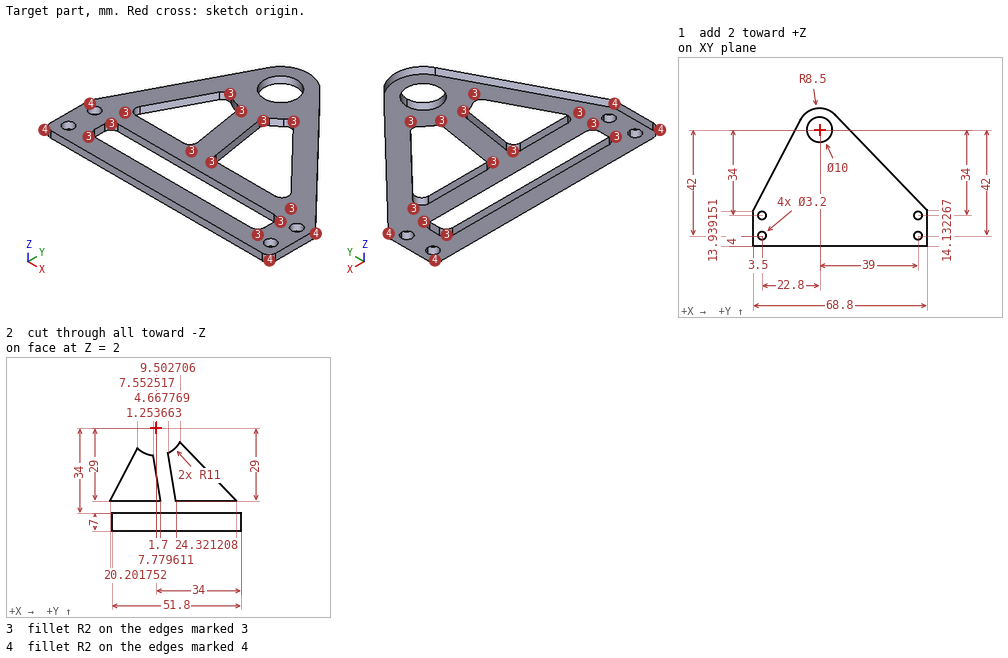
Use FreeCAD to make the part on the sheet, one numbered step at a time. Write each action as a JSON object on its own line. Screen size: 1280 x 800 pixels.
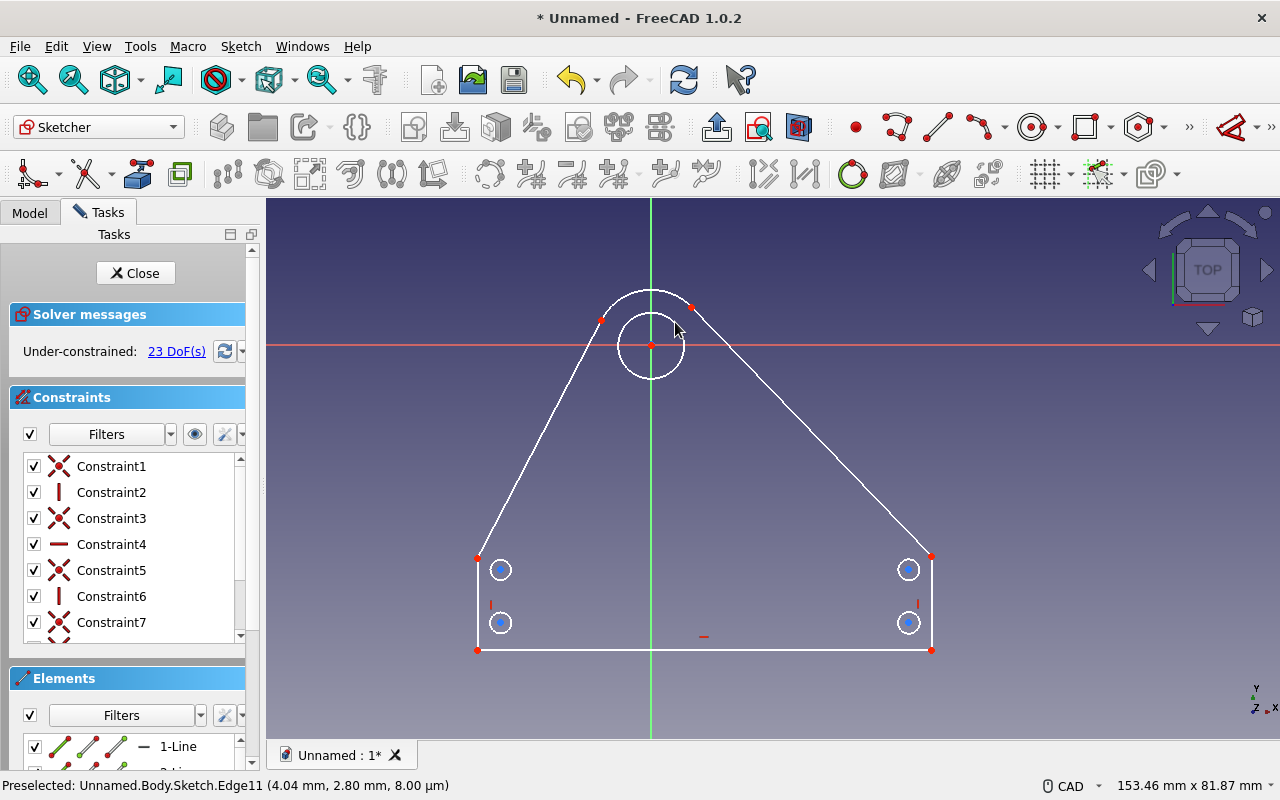
{"action": "left_click", "coordinate": [564, 392]}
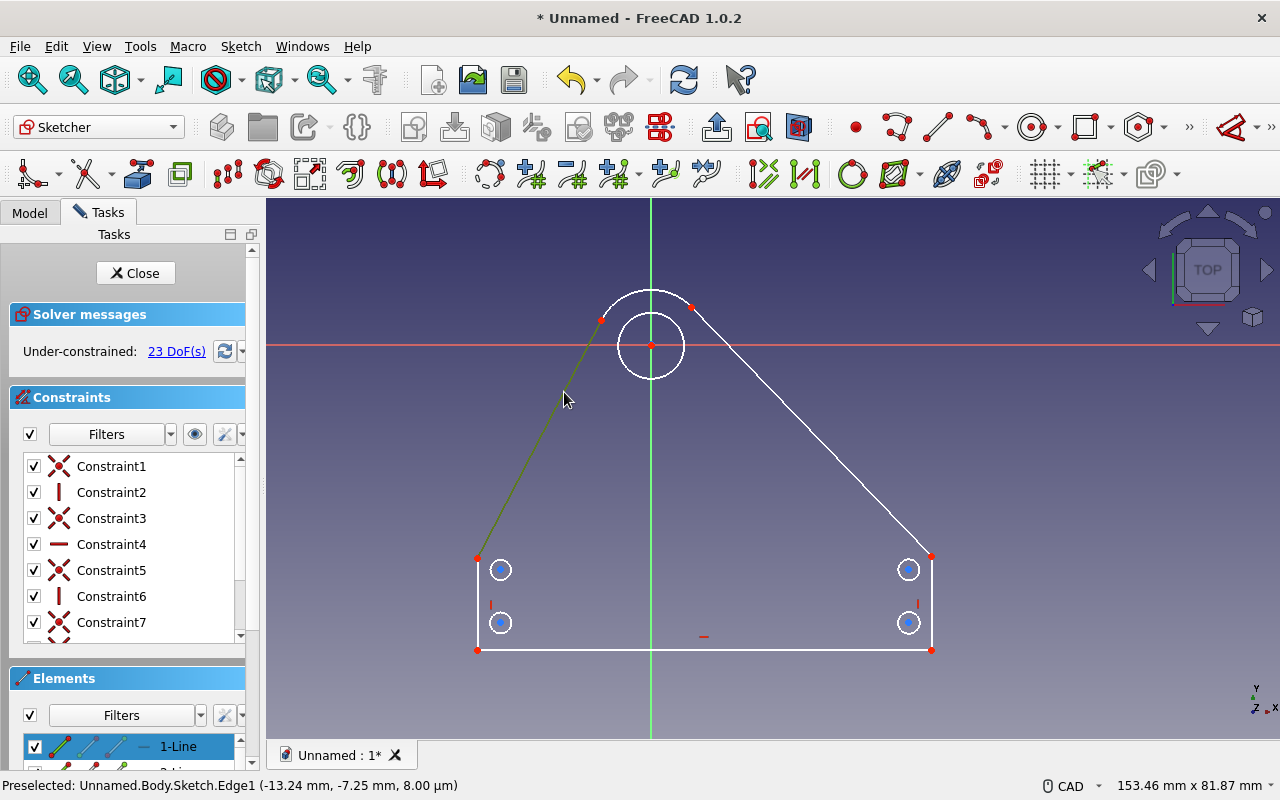
{"action": "left_click", "coordinate": [664, 291]}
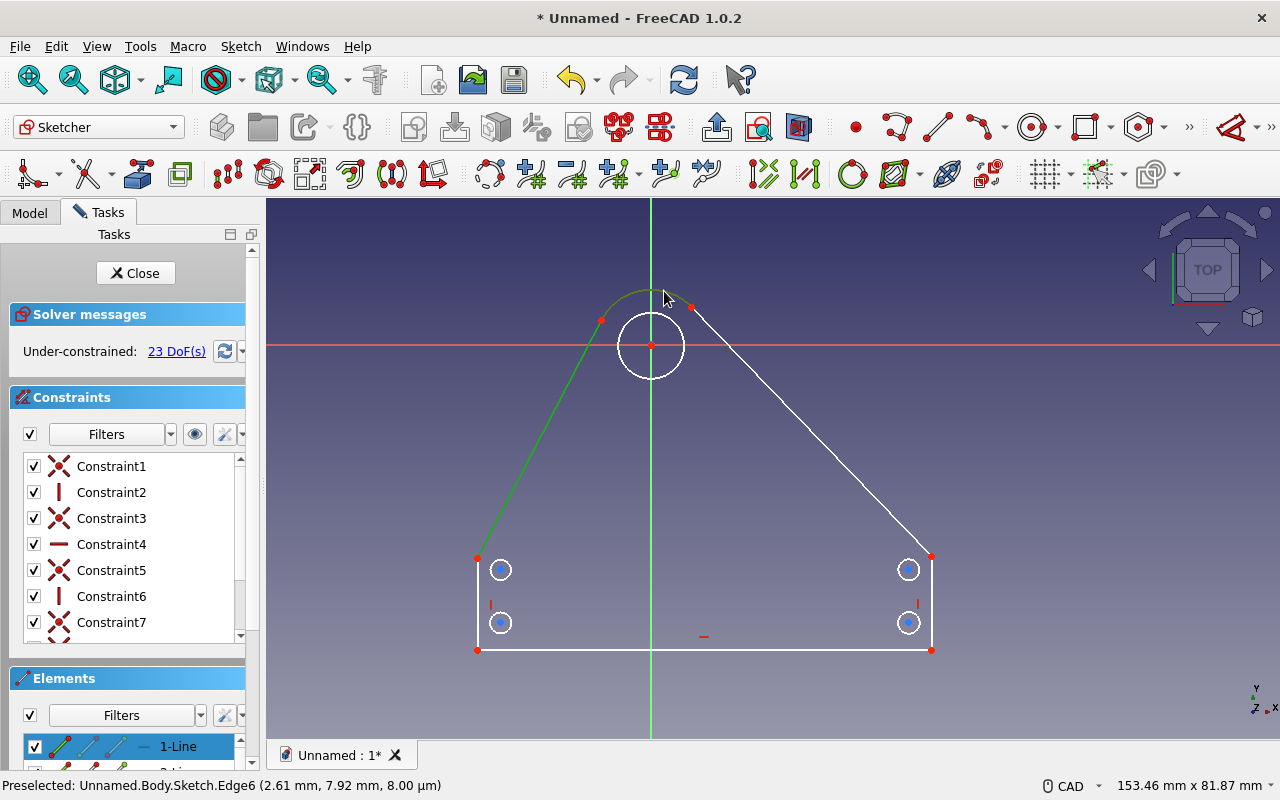
{"action": "key", "text": "t"}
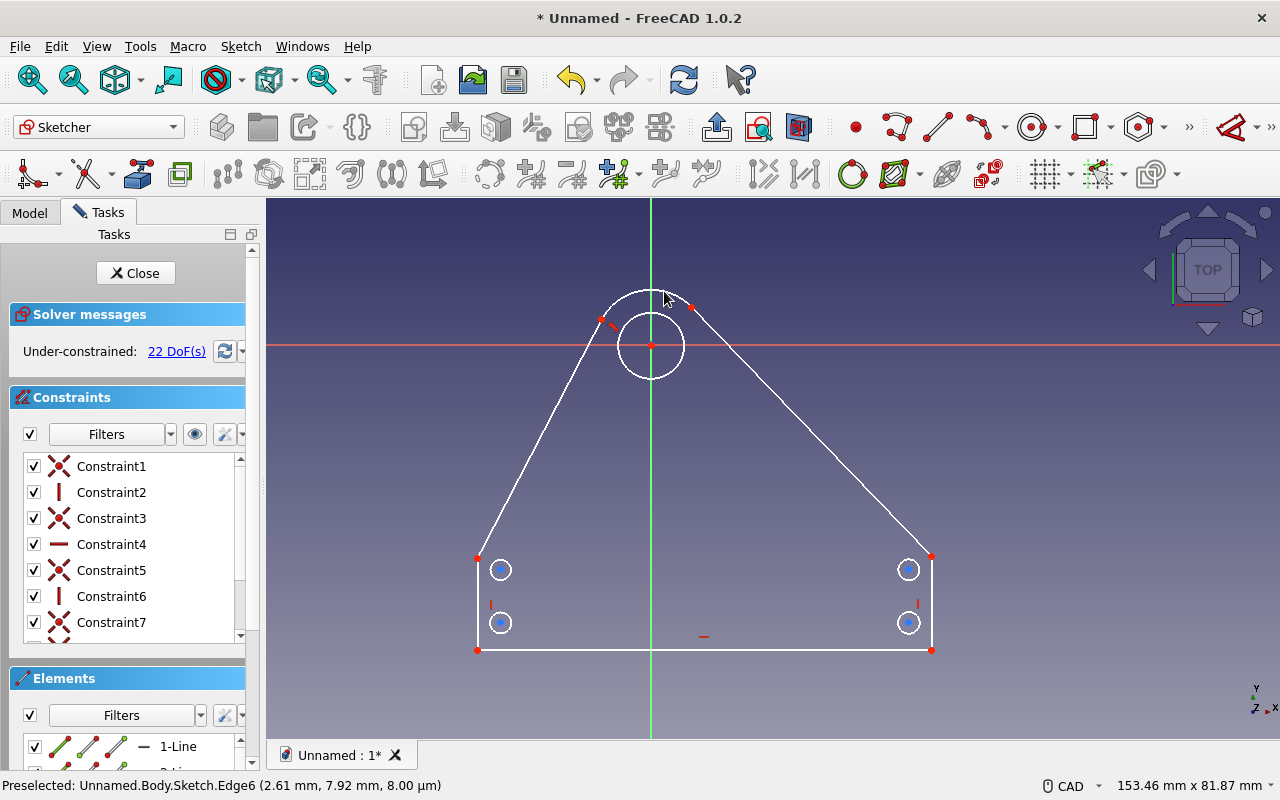
{"action": "left_click", "coordinate": [860, 481]}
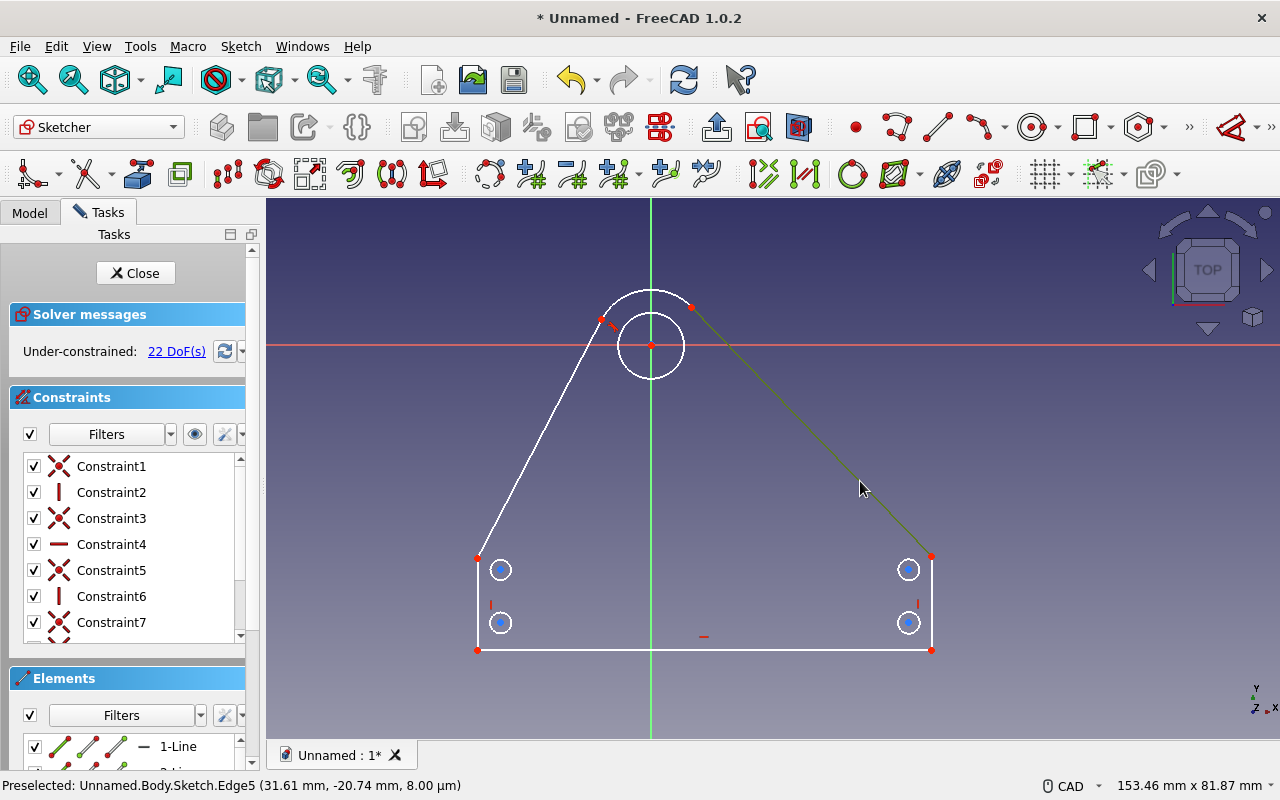
{"action": "left_click", "coordinate": [664, 291]}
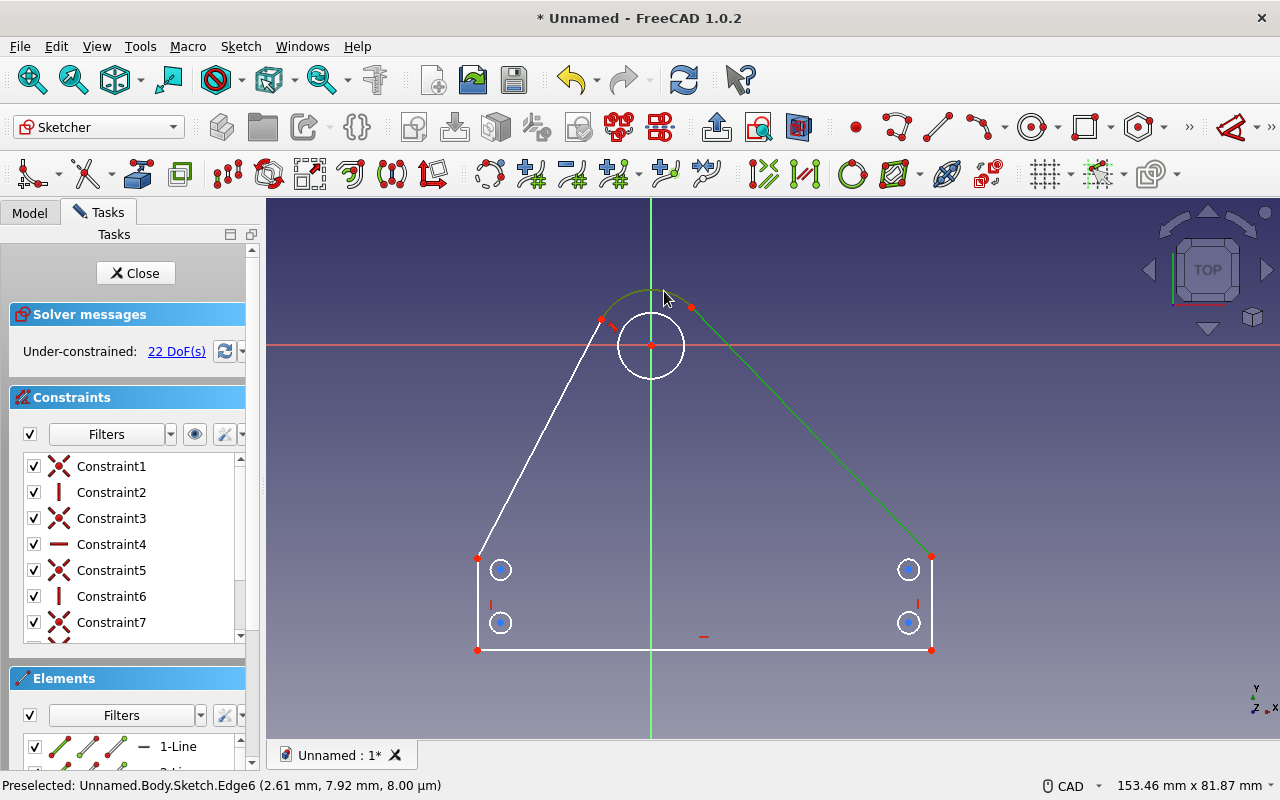
{"action": "key", "text": "t"}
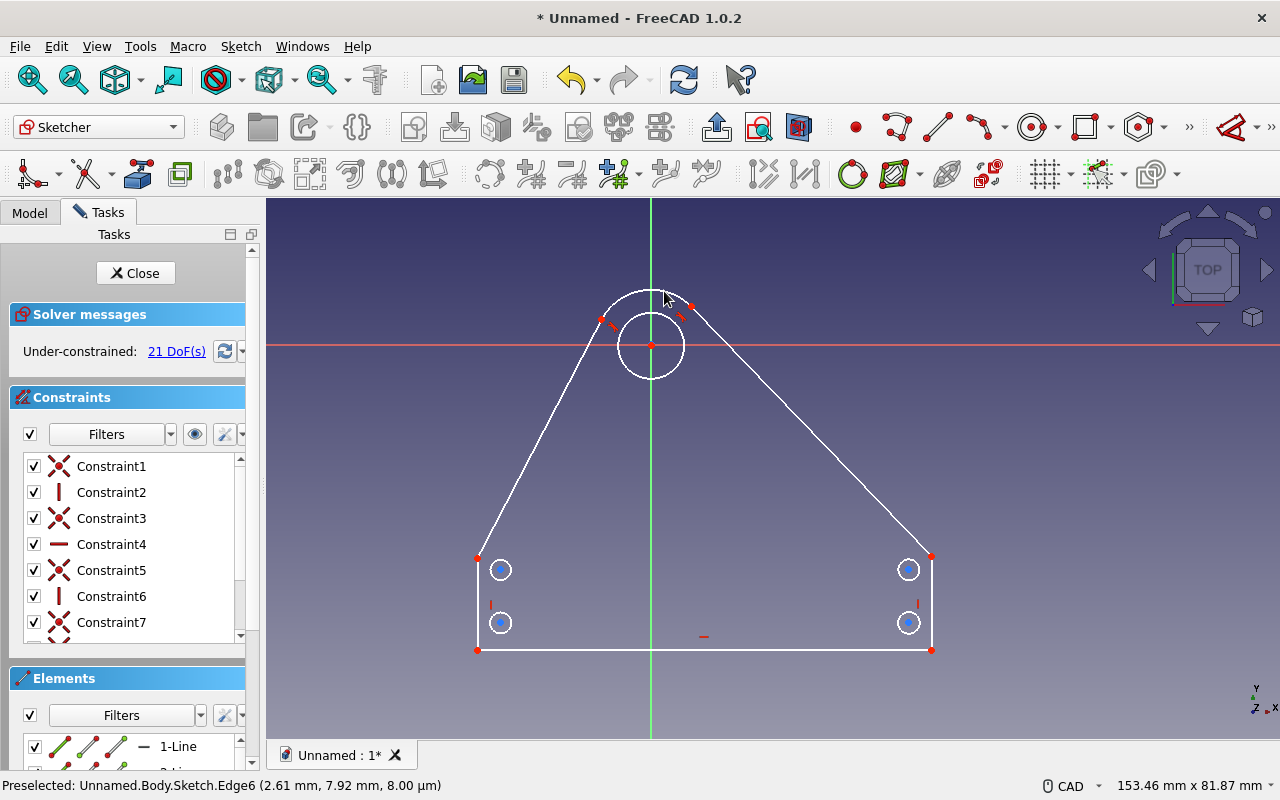
{"action": "scroll", "coordinate": [651, 345], "scroll_direction": "up", "scroll_amount": 7}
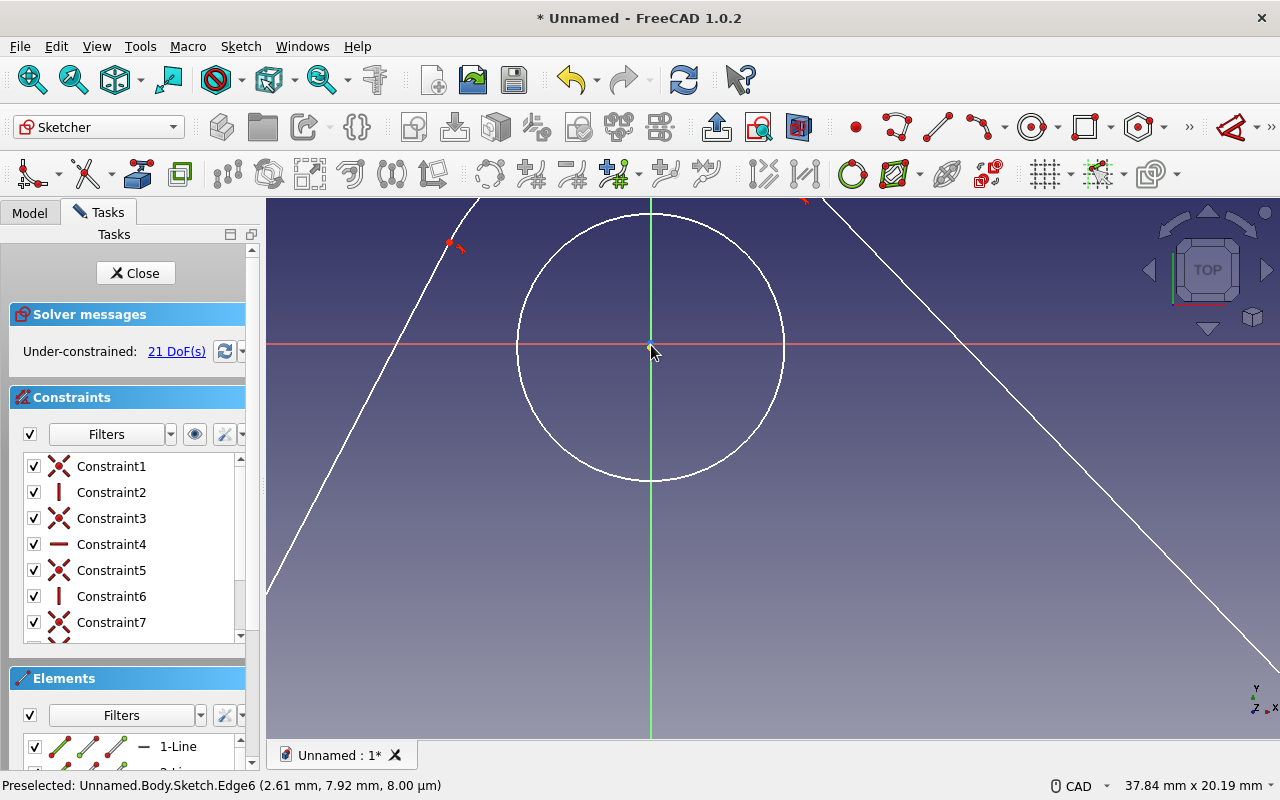
{"action": "left_click_drag", "start_coordinate": [641, 334], "coordinate": [661, 357]}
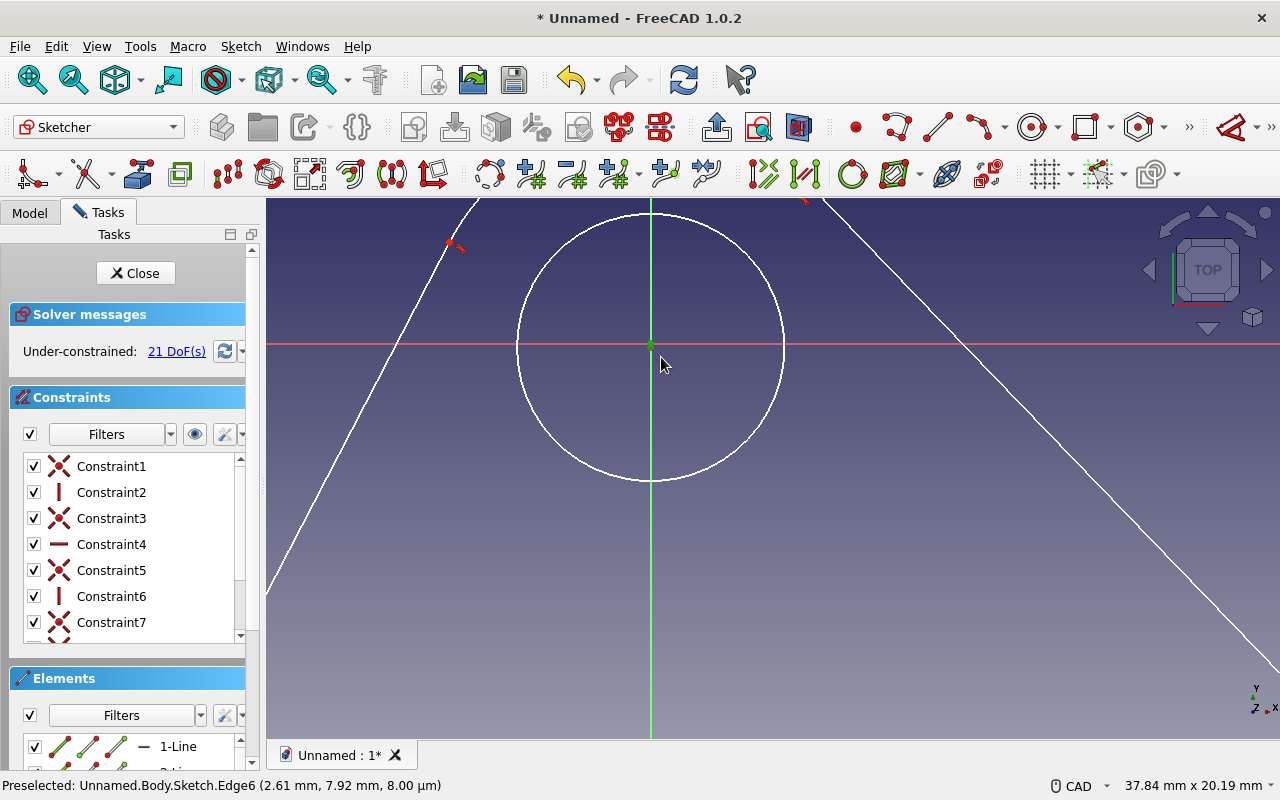
{"action": "key", "text": "c"}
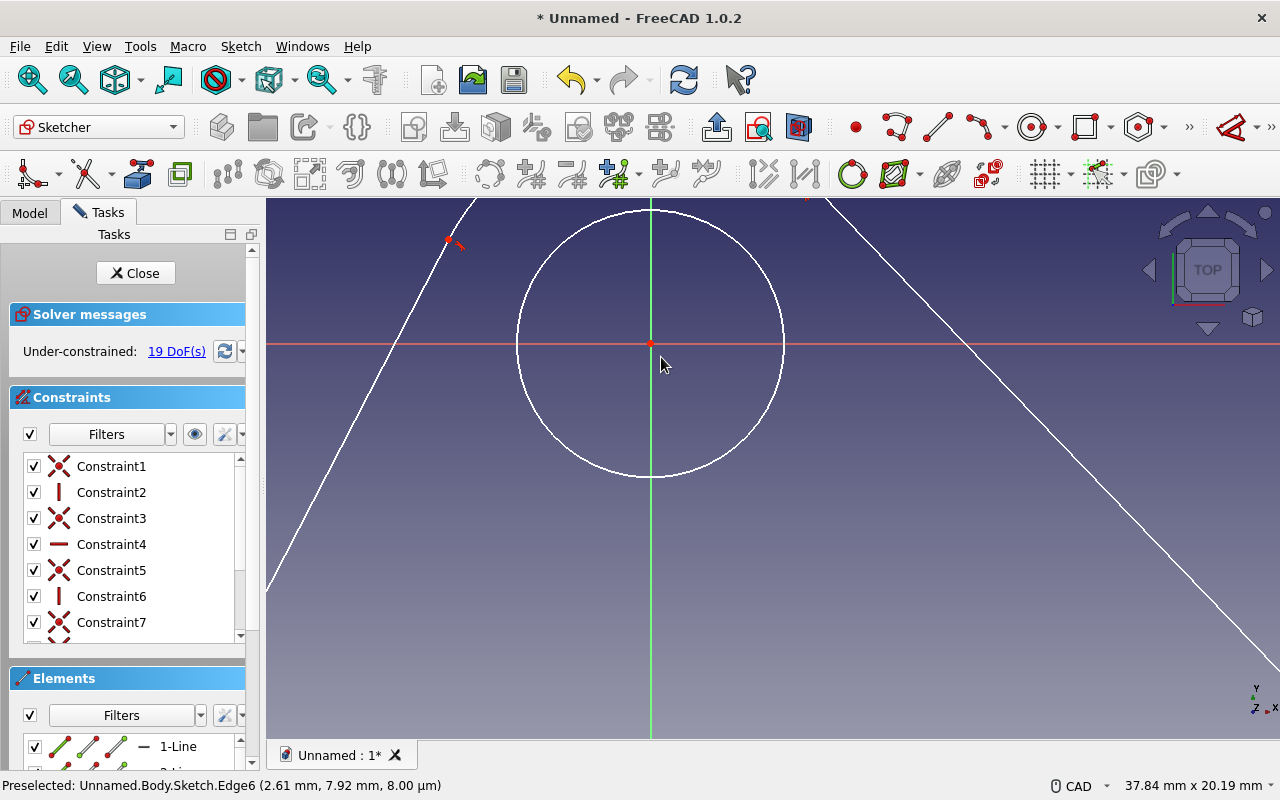
{"action": "scroll", "coordinate": [651, 344], "scroll_direction": "down", "scroll_amount": 7}